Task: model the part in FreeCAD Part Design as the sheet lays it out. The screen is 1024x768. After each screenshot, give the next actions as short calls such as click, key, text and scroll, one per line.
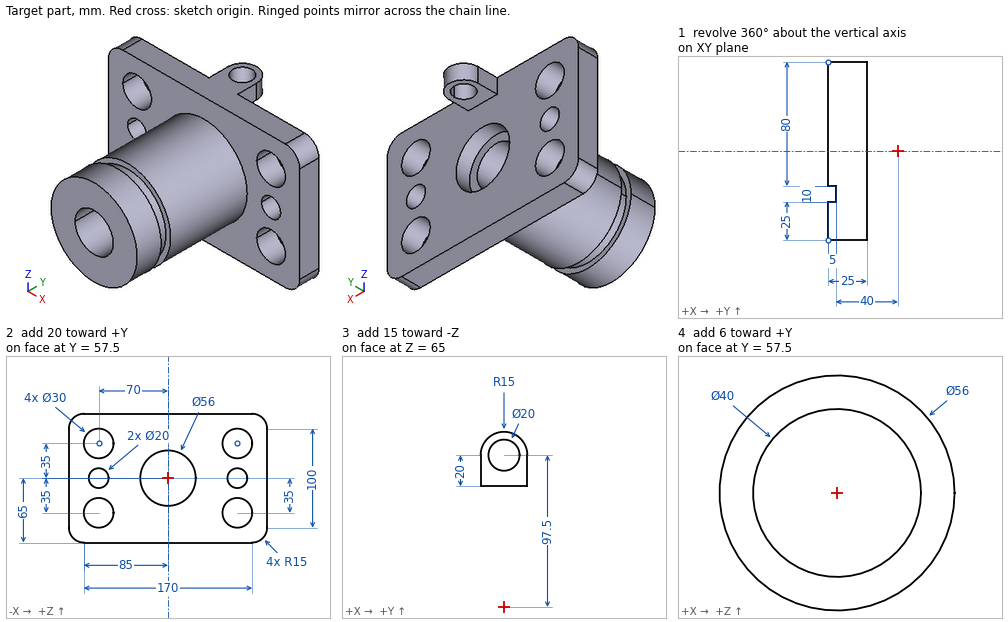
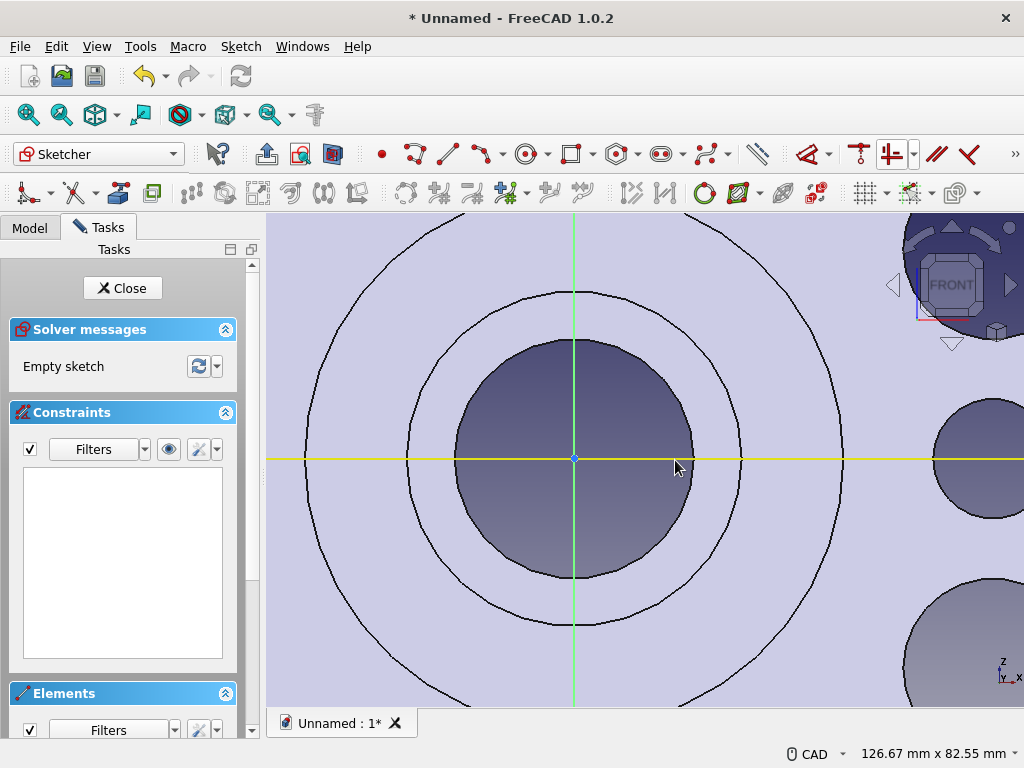
click(526, 154)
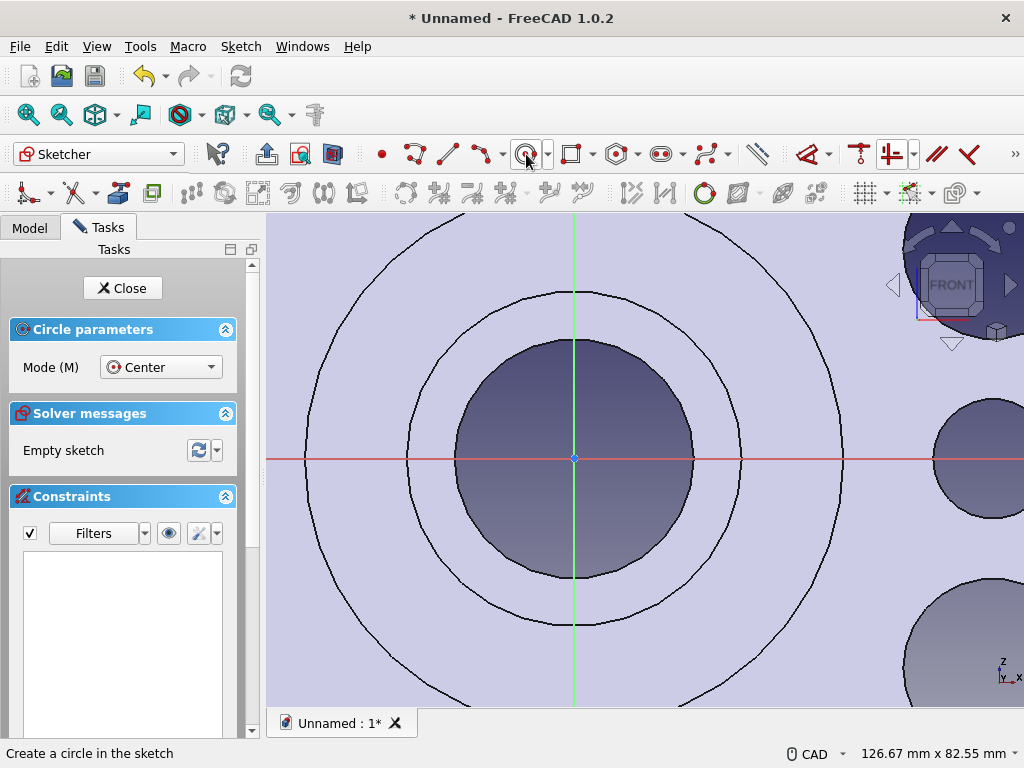
click(574, 459)
move(693, 340)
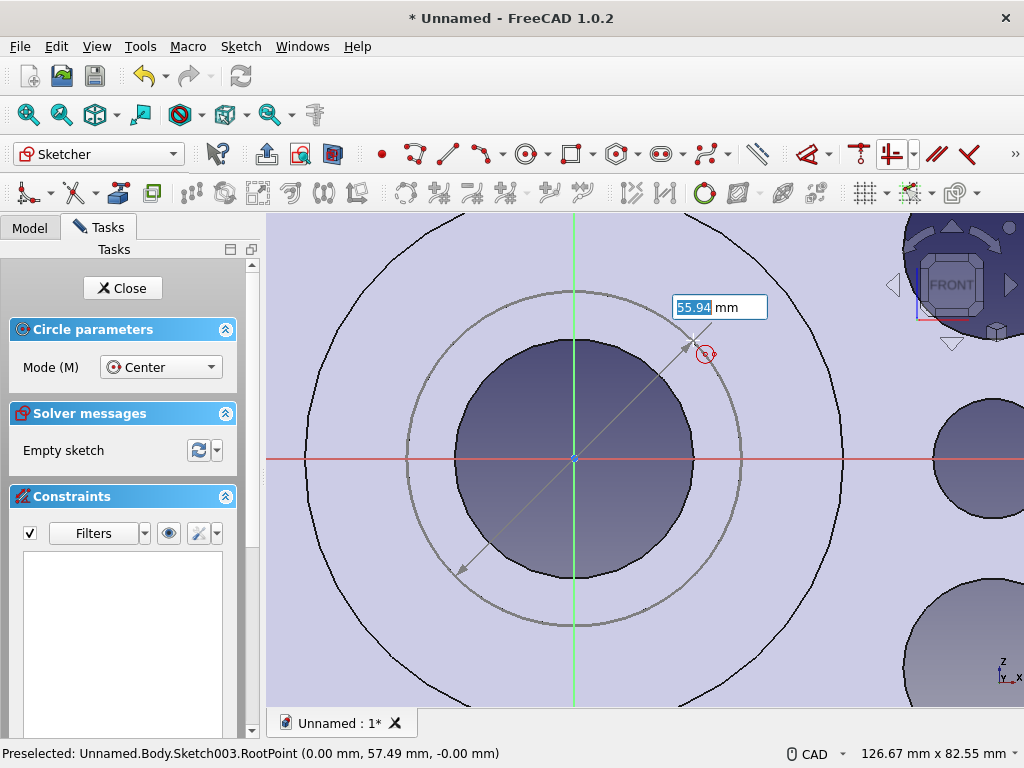
text(56)
key(Return)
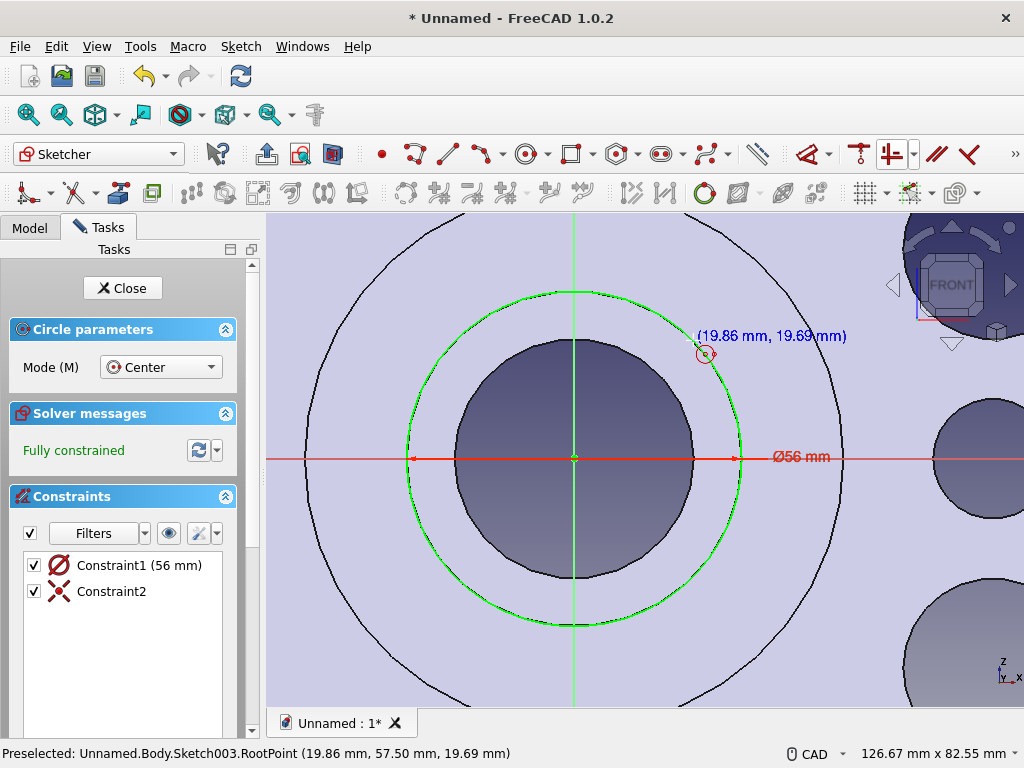
click(574, 459)
move(659, 374)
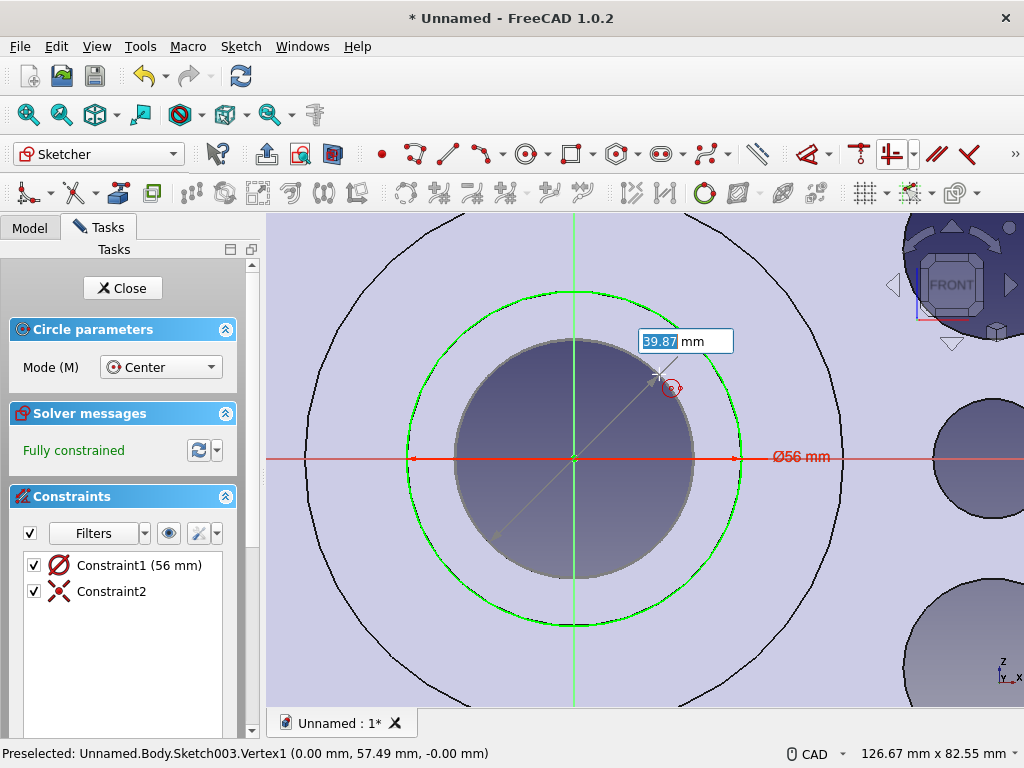
text(40)
key(Return)
key(Escape)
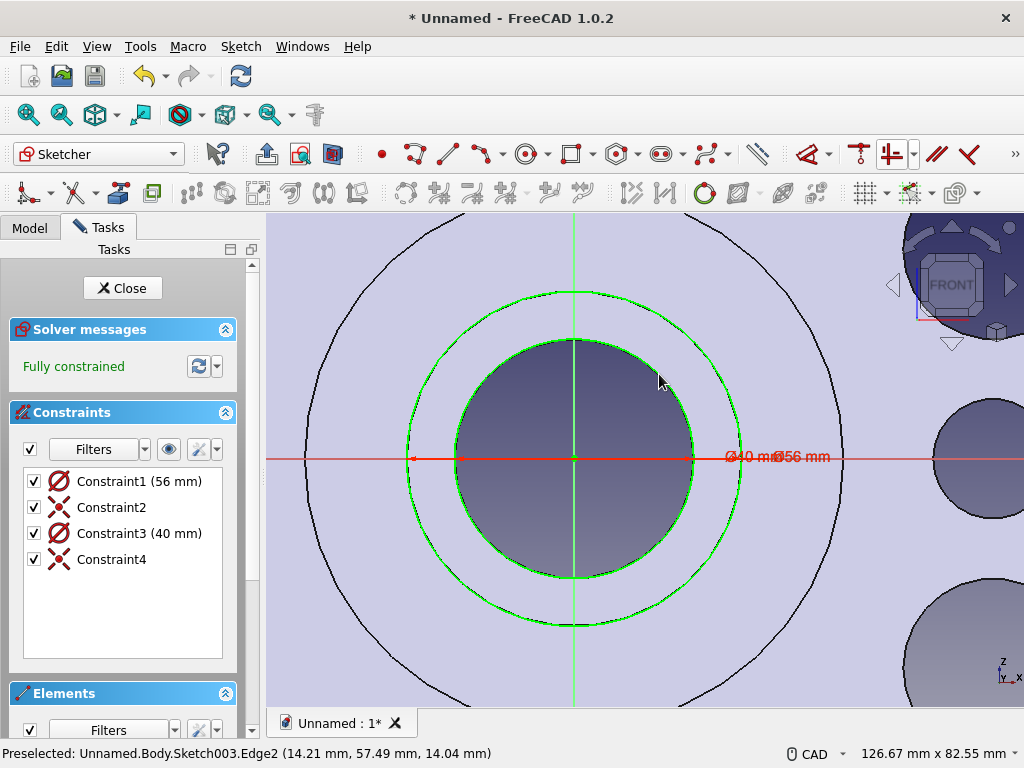
click(123, 288)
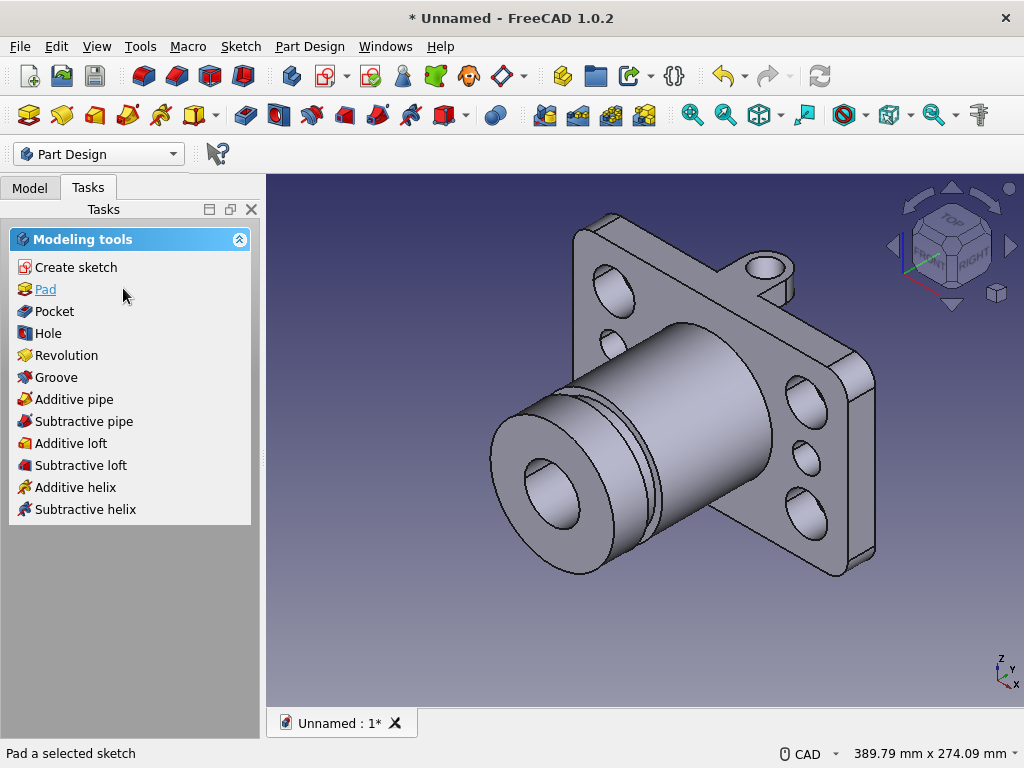
click(29, 116)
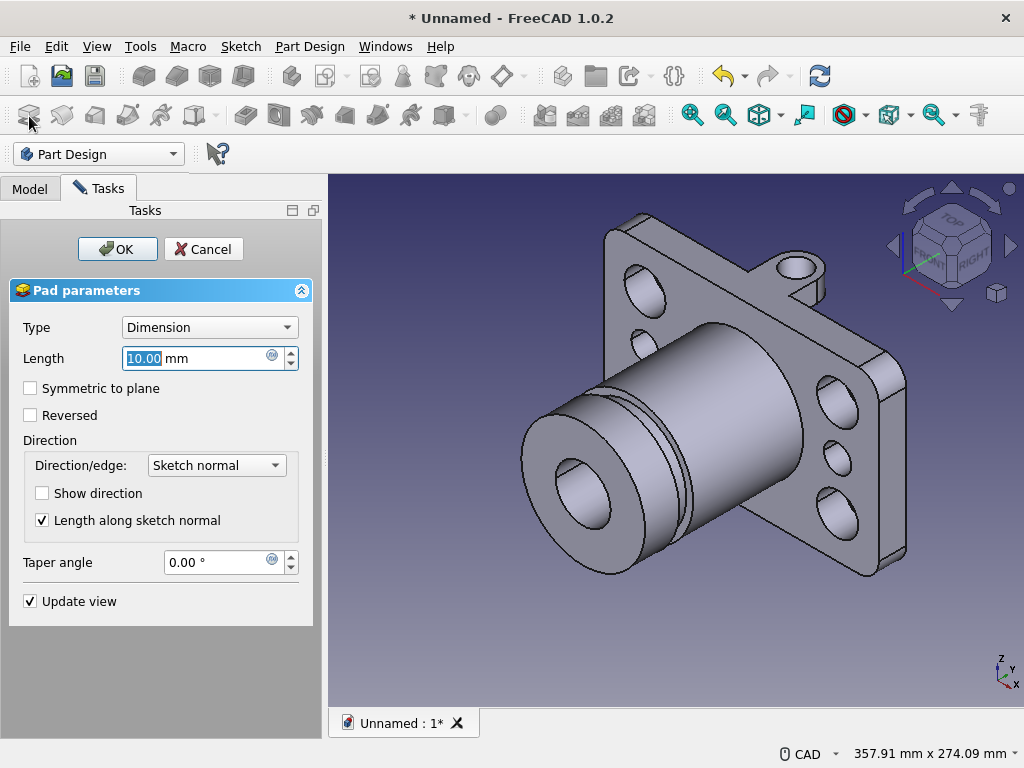
text(6)
key(Tab)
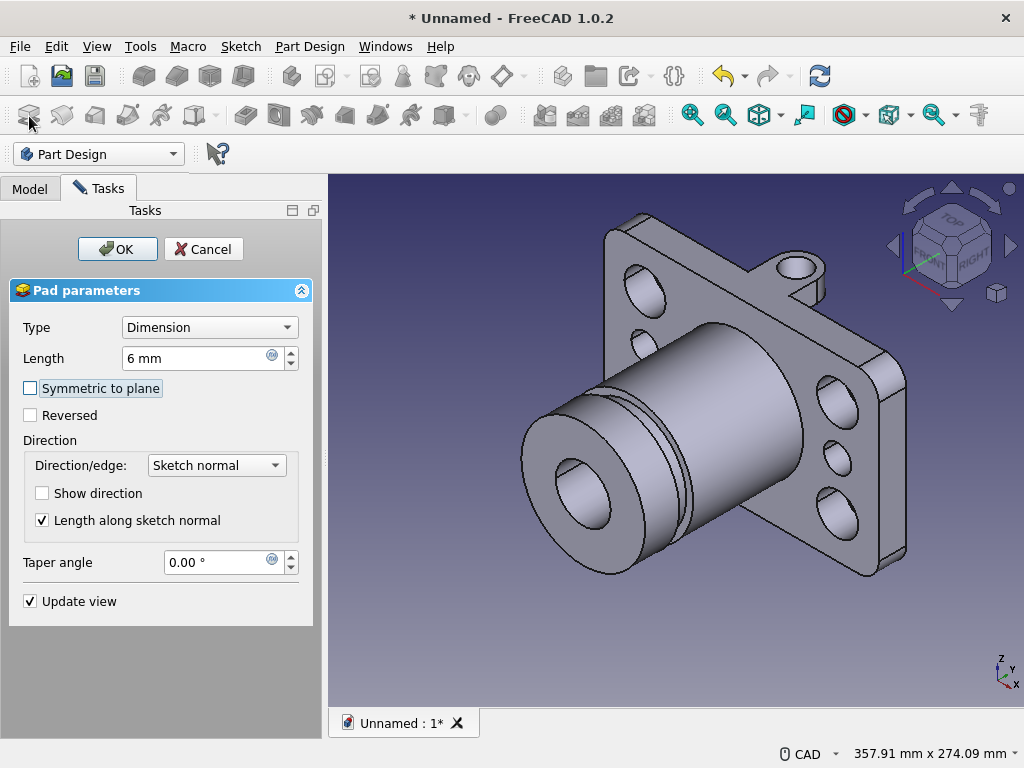
click(31, 415)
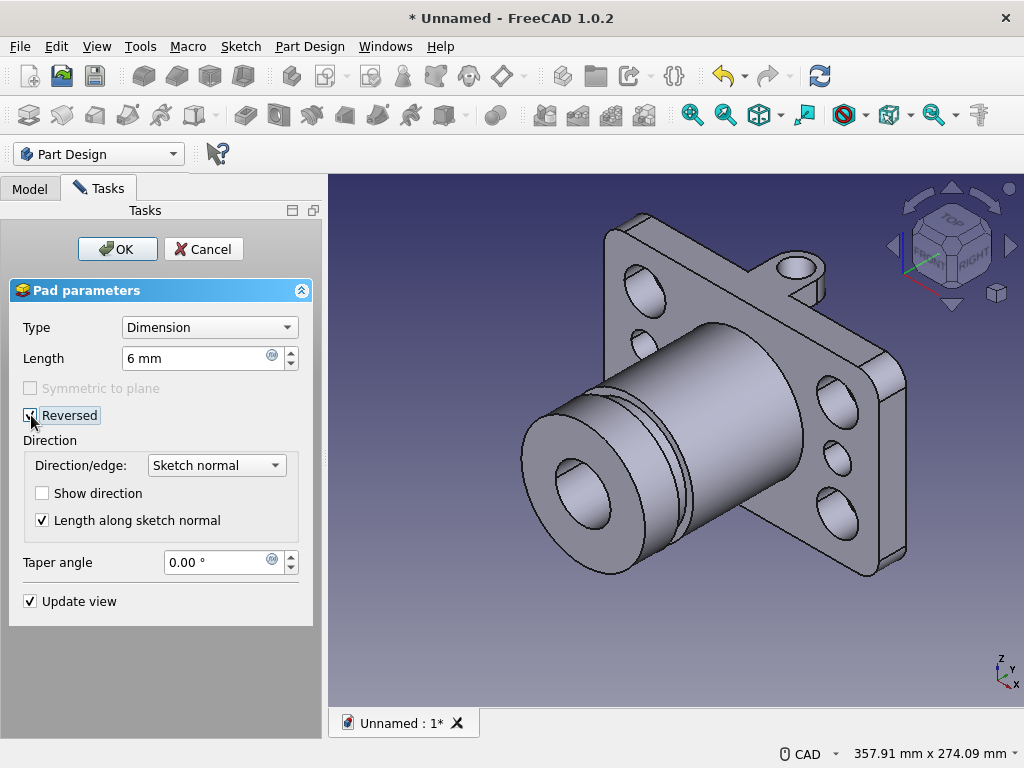
click(118, 249)